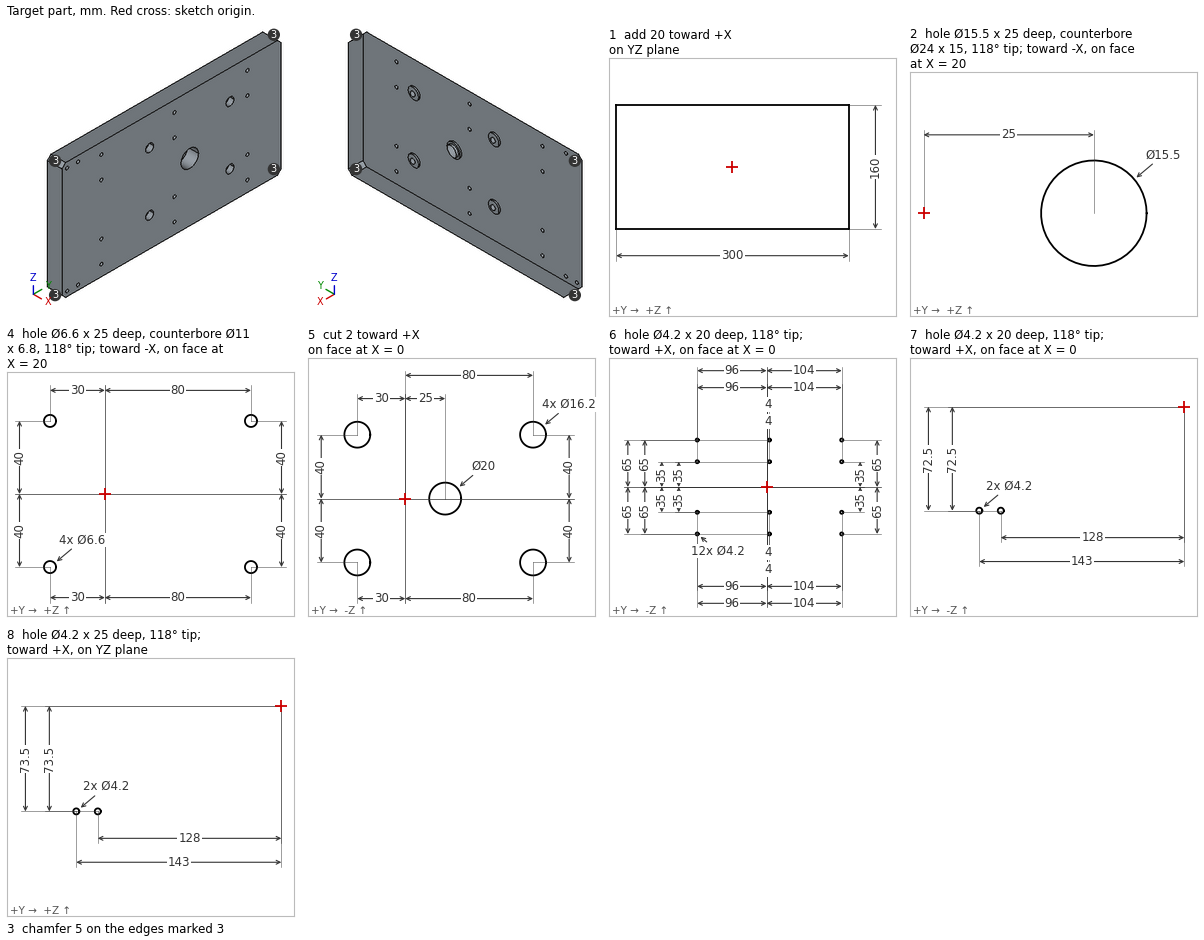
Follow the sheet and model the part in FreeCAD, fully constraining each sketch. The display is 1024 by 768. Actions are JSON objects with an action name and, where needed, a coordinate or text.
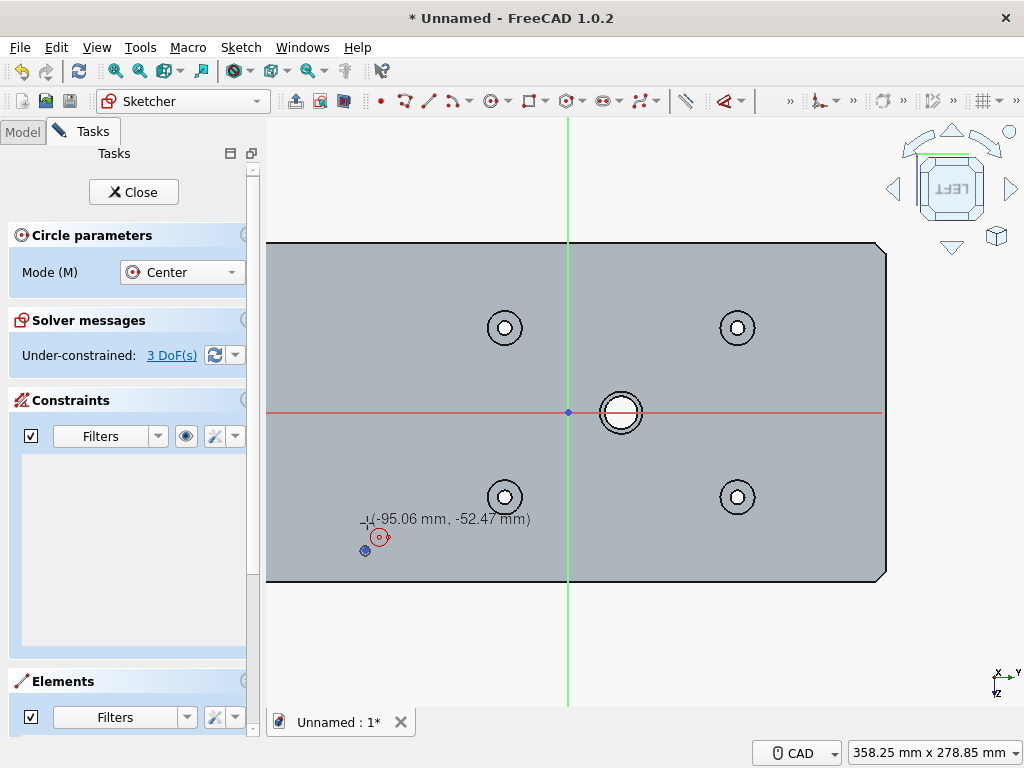
{"action": "left_click", "coordinate": [365, 487]}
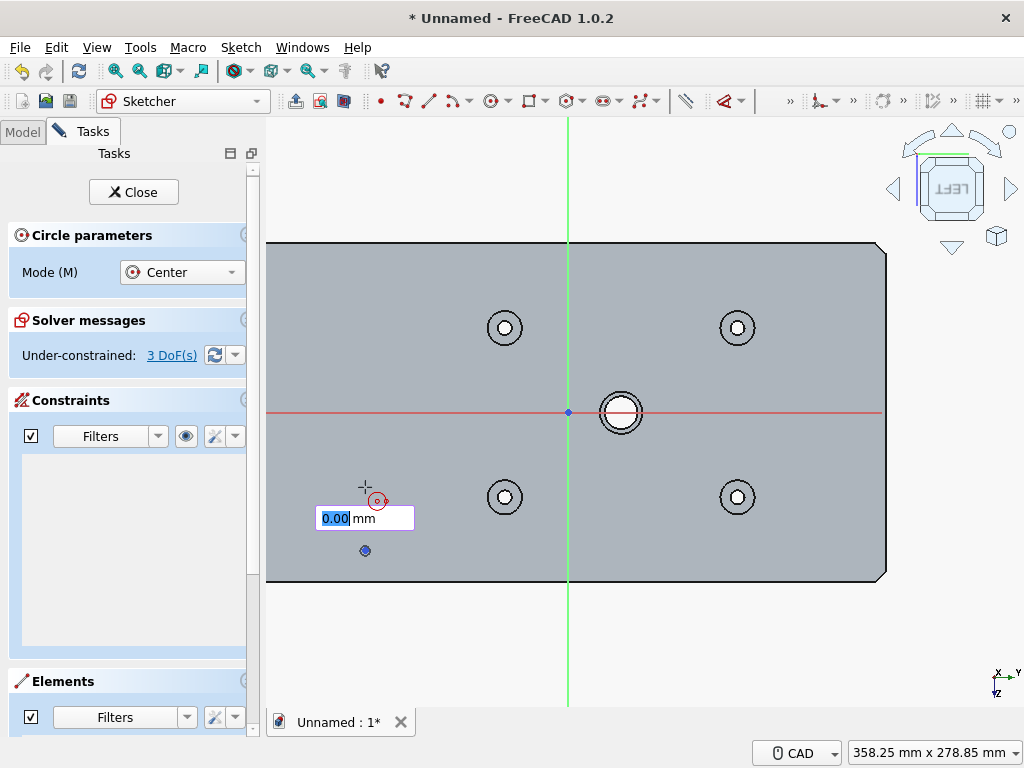
{"action": "scroll", "coordinate": [368, 484], "scroll_direction": "up", "scroll_amount": 7}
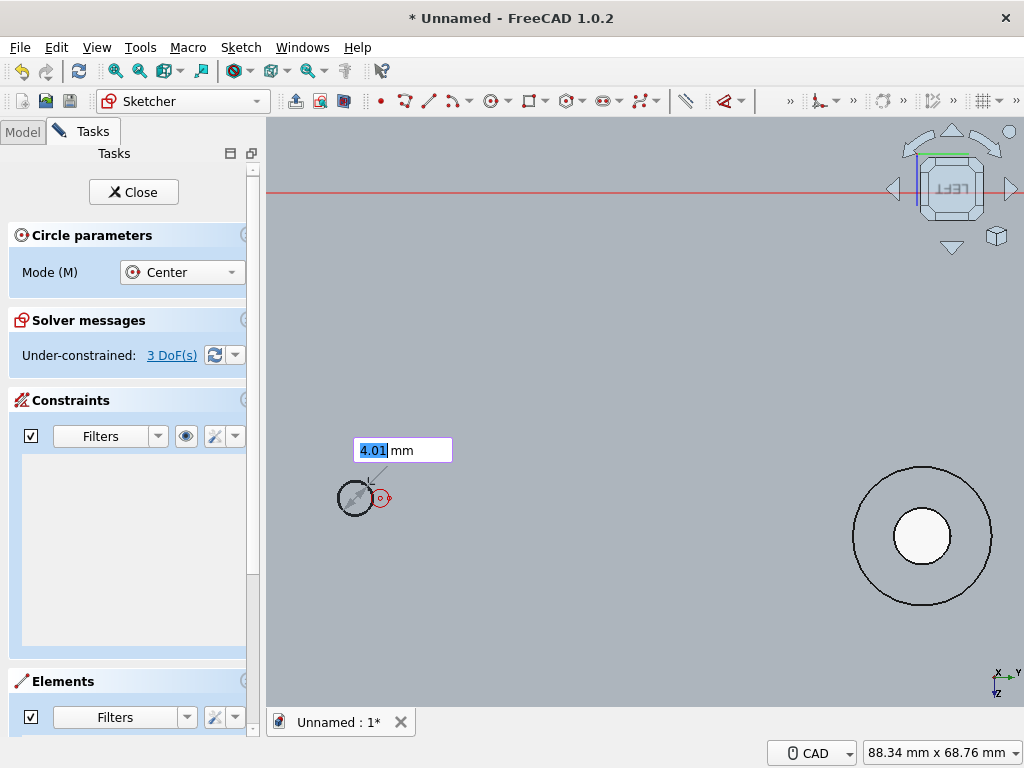
{"action": "left_click", "coordinate": [369, 481]}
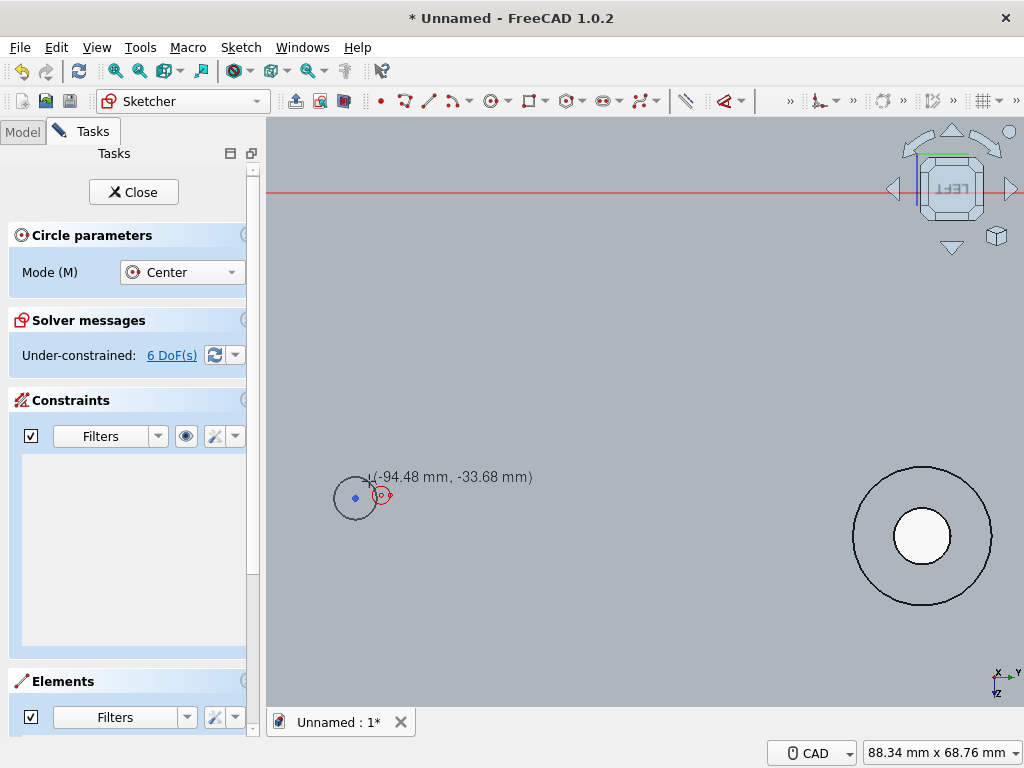
{"action": "scroll", "coordinate": [368, 484], "scroll_direction": "down", "scroll_amount": 7}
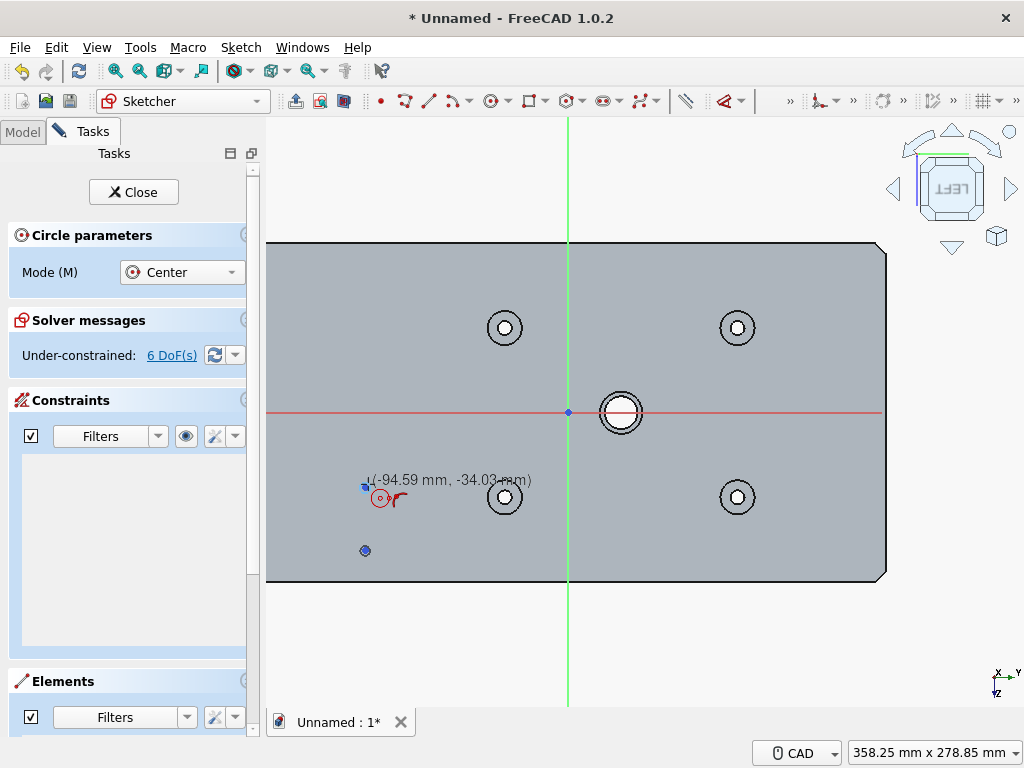
{"action": "scroll", "coordinate": [577, 550], "scroll_direction": "up", "scroll_amount": 9}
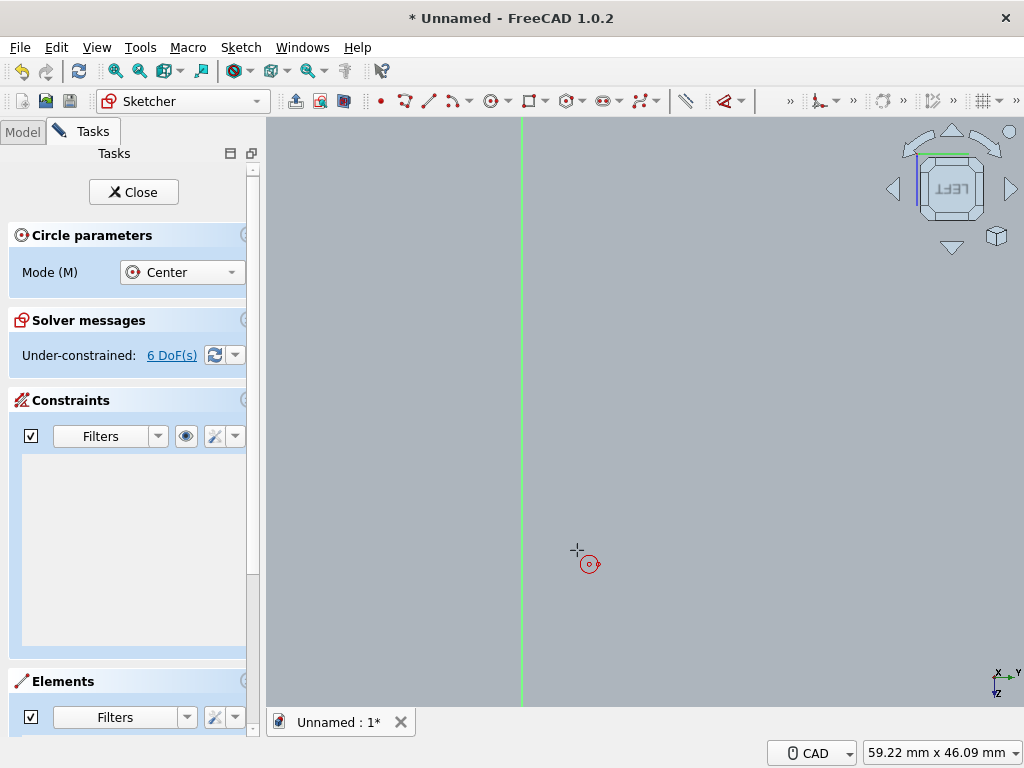
{"action": "scroll", "coordinate": [577, 550], "scroll_direction": "down", "scroll_amount": 9}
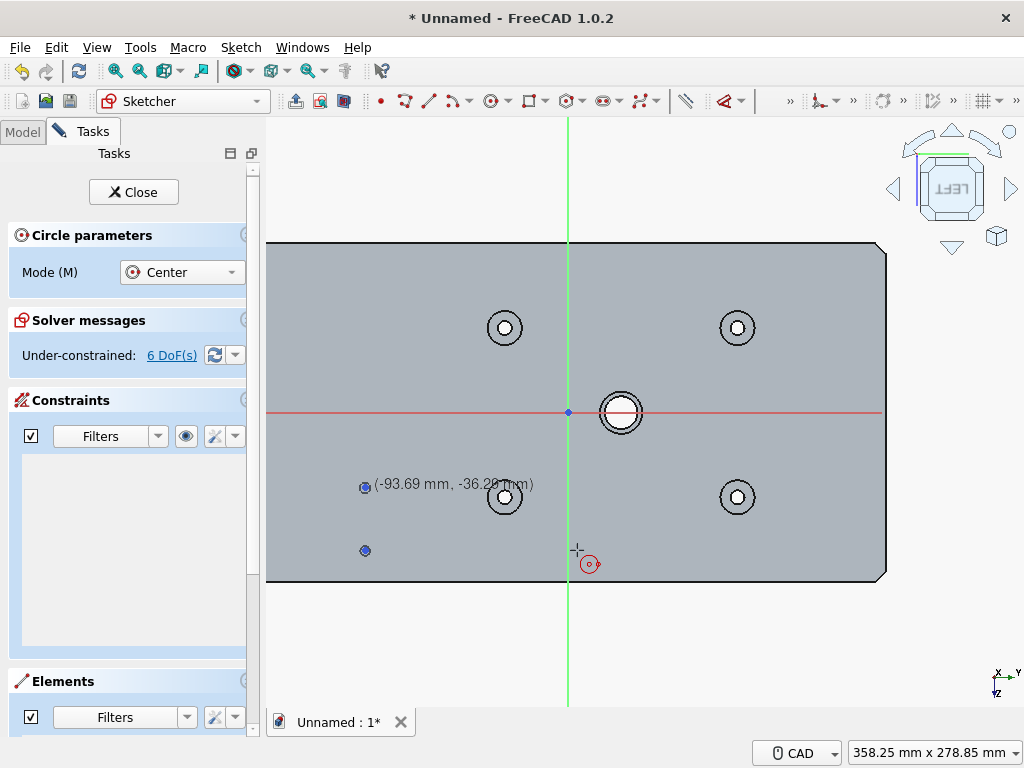
{"action": "scroll", "coordinate": [577, 550], "scroll_direction": "up", "scroll_amount": 4}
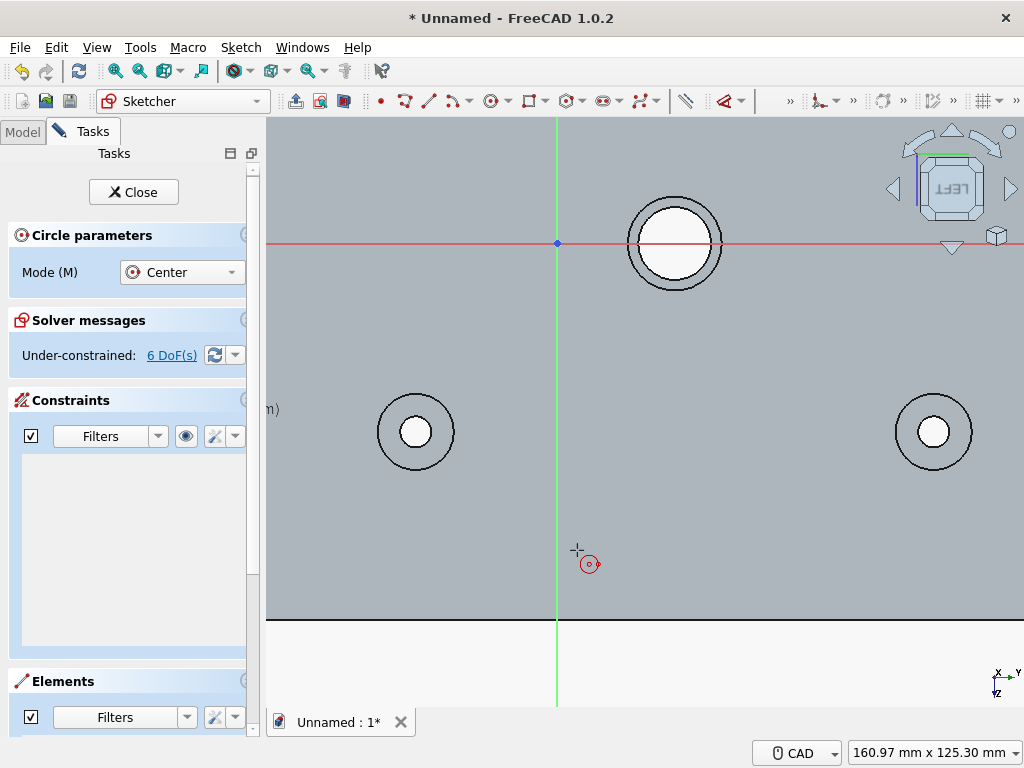
{"action": "left_click", "coordinate": [576, 550]}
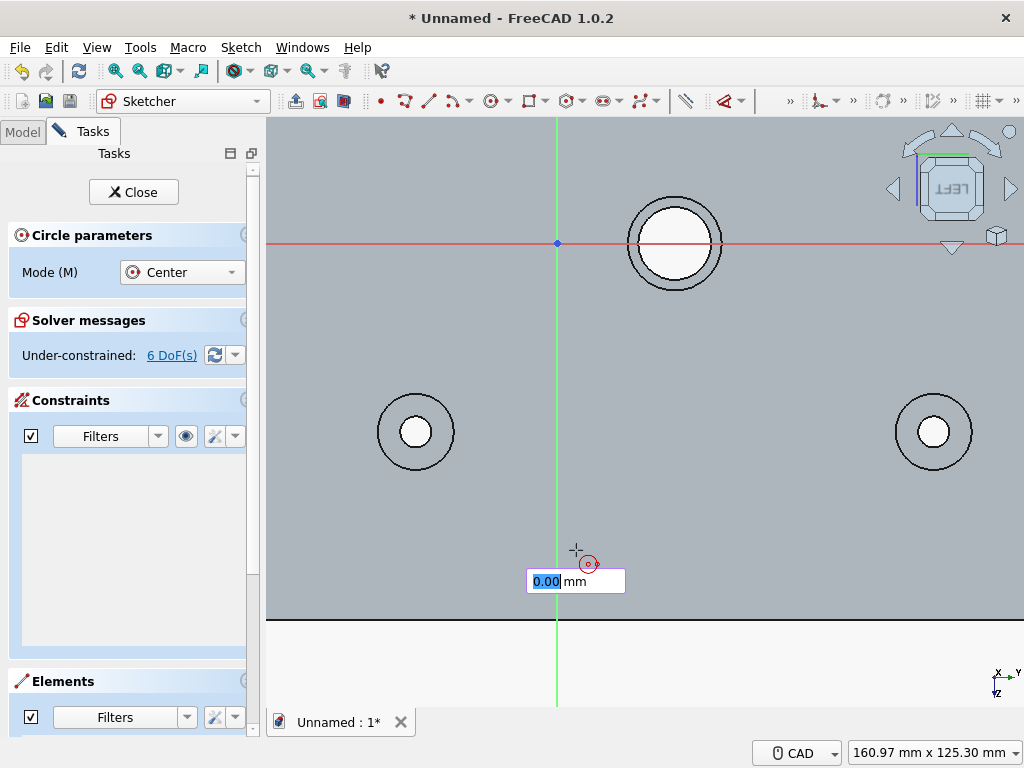
{"action": "scroll", "coordinate": [583, 543], "scroll_direction": "up", "scroll_amount": 3}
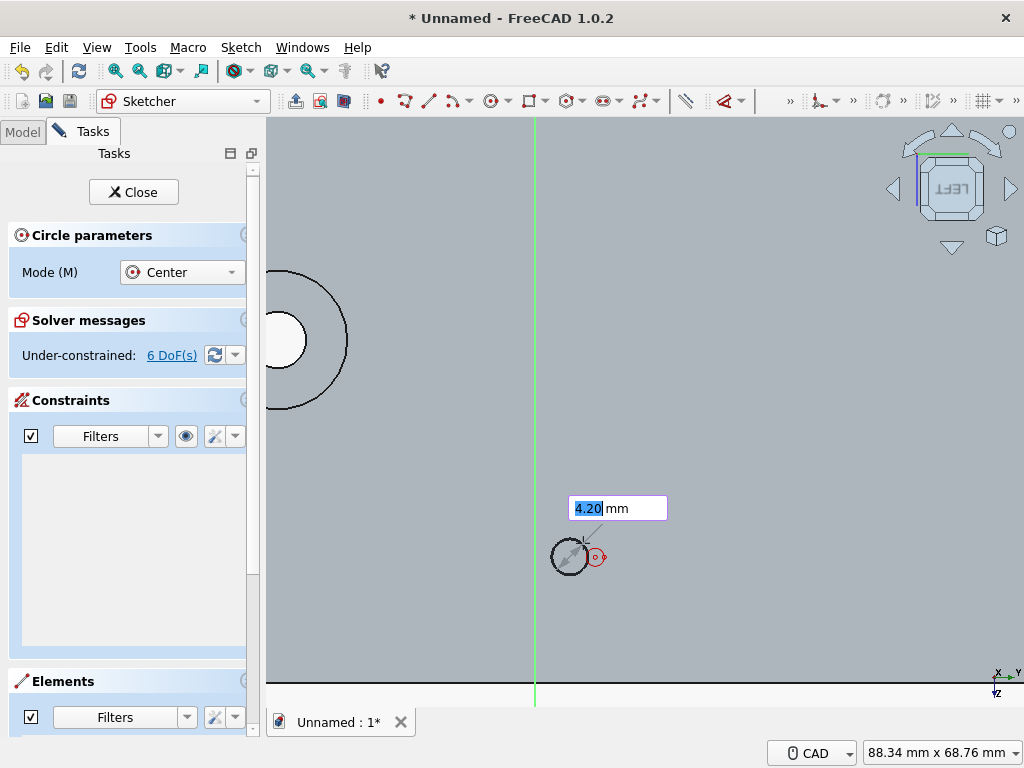
{"action": "left_click", "coordinate": [582, 542]}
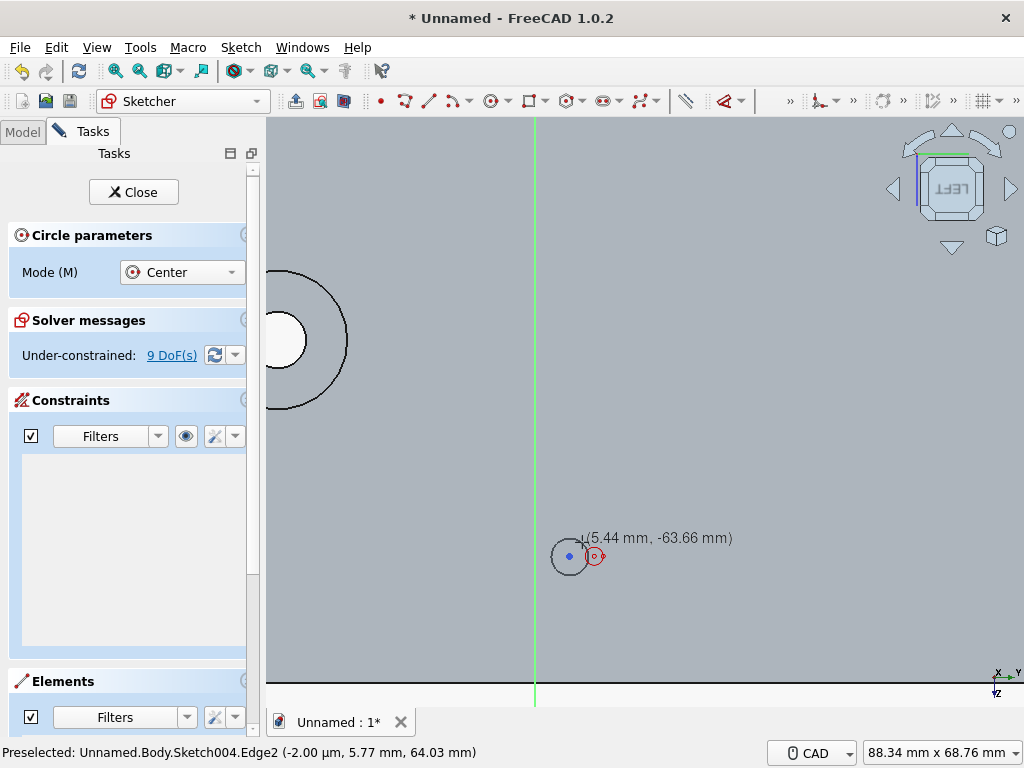
{"action": "scroll", "coordinate": [570, 297], "scroll_direction": "up", "scroll_amount": 2}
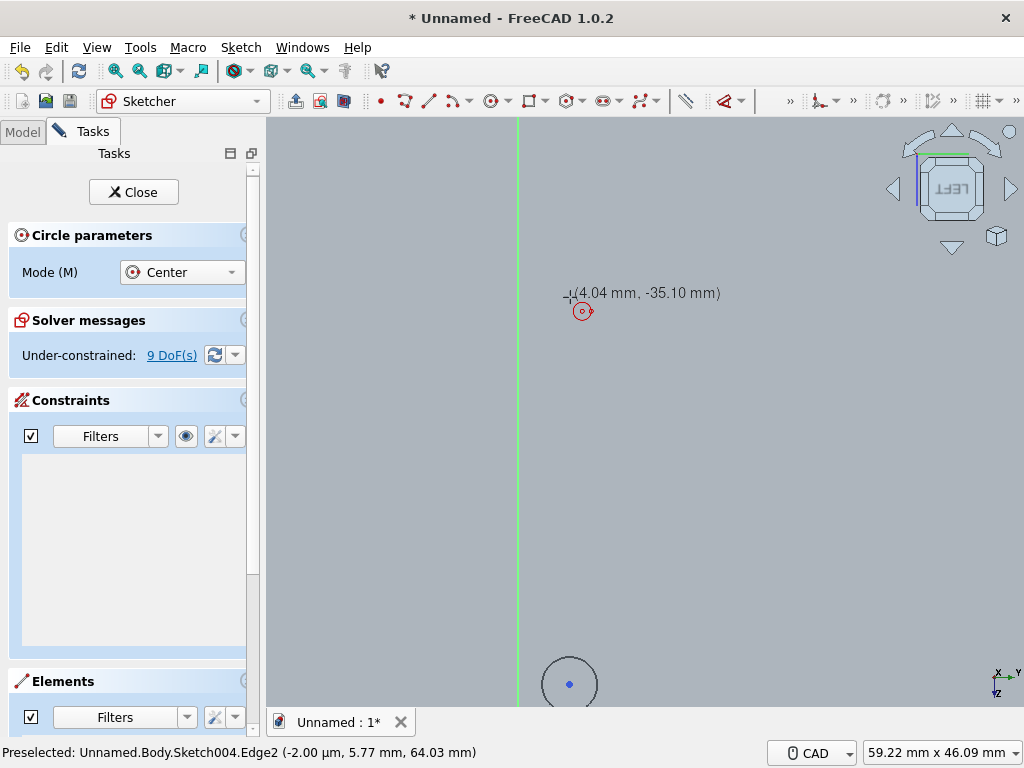
{"action": "scroll", "coordinate": [578, 523], "scroll_direction": "down", "scroll_amount": 9}